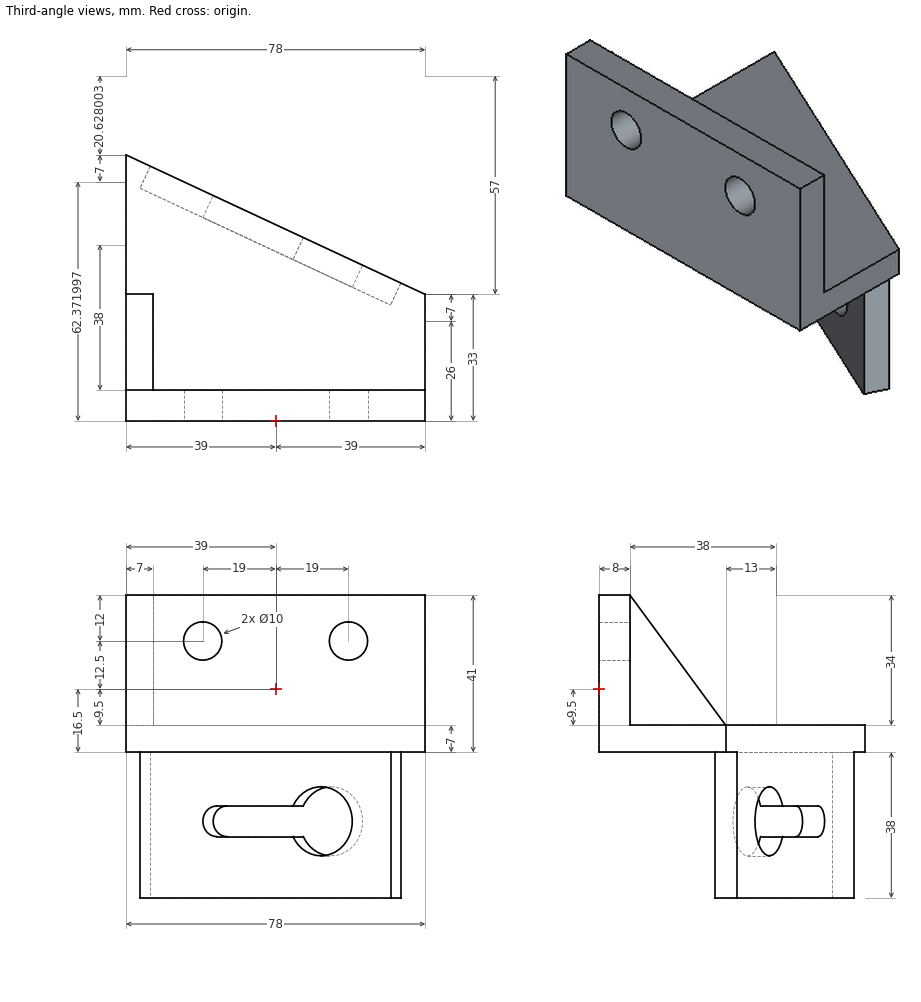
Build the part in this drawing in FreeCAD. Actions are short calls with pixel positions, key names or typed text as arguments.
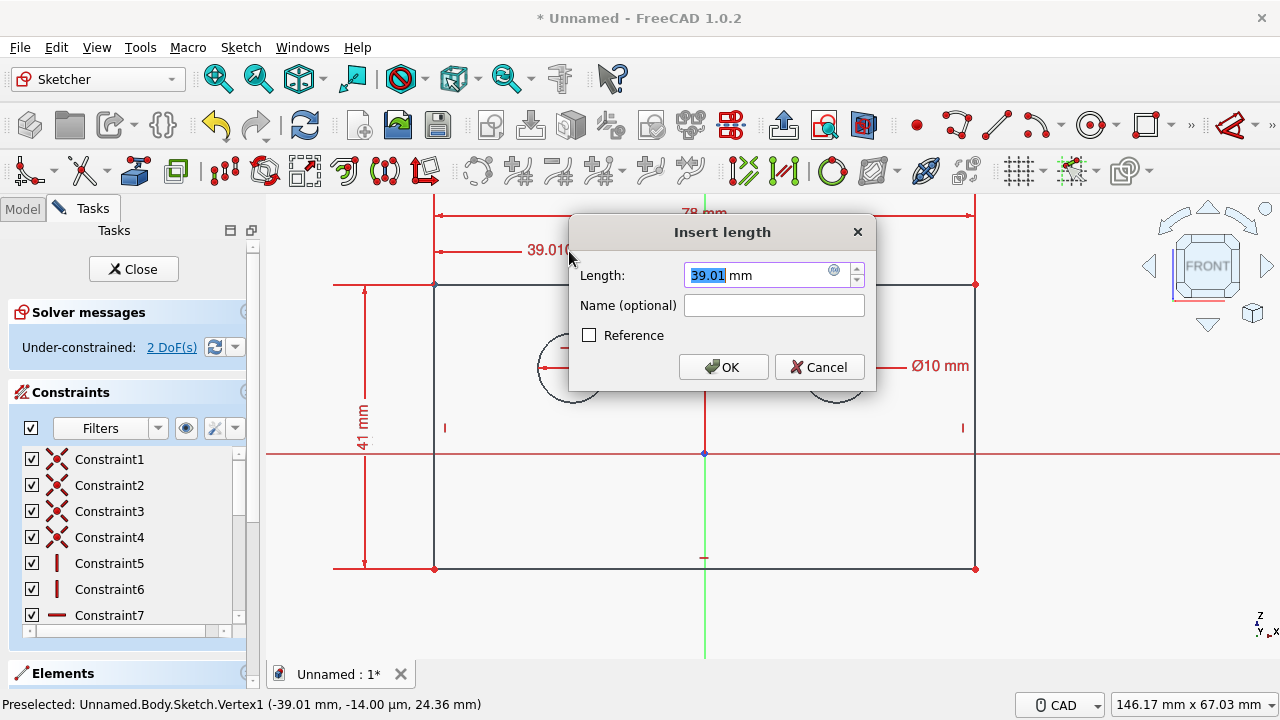
text(39)
key(Return)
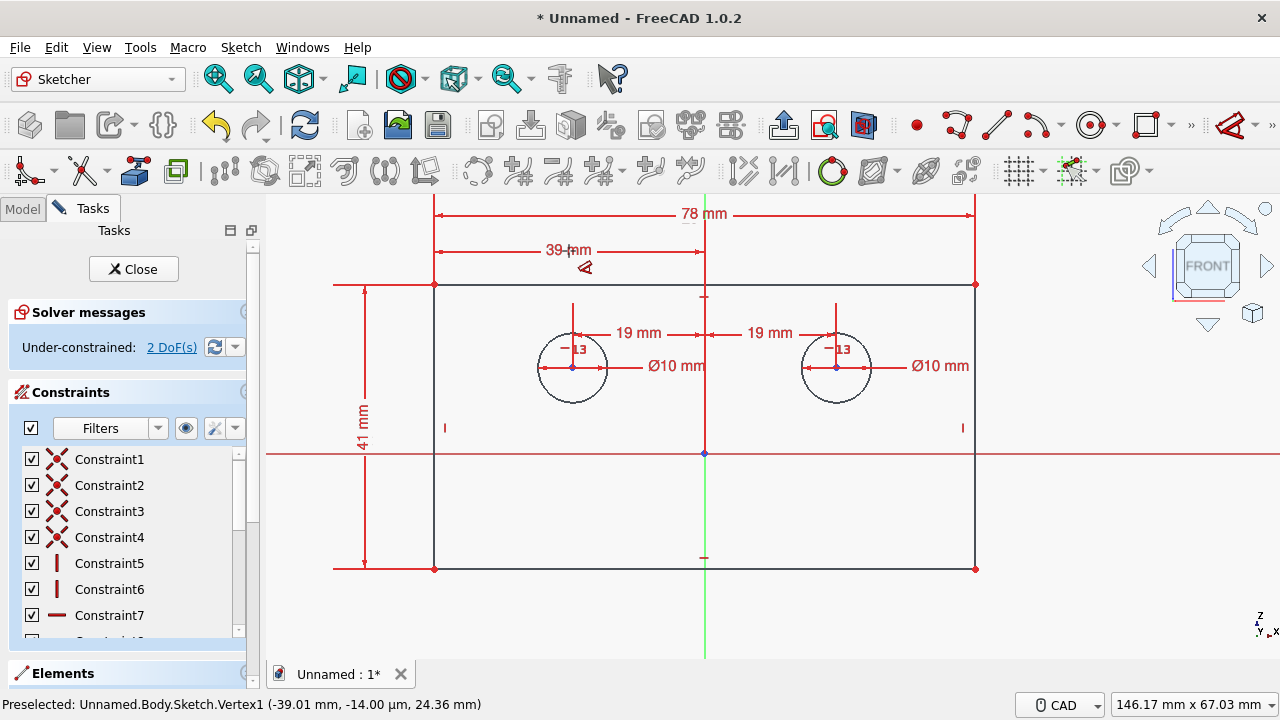
click(434, 285)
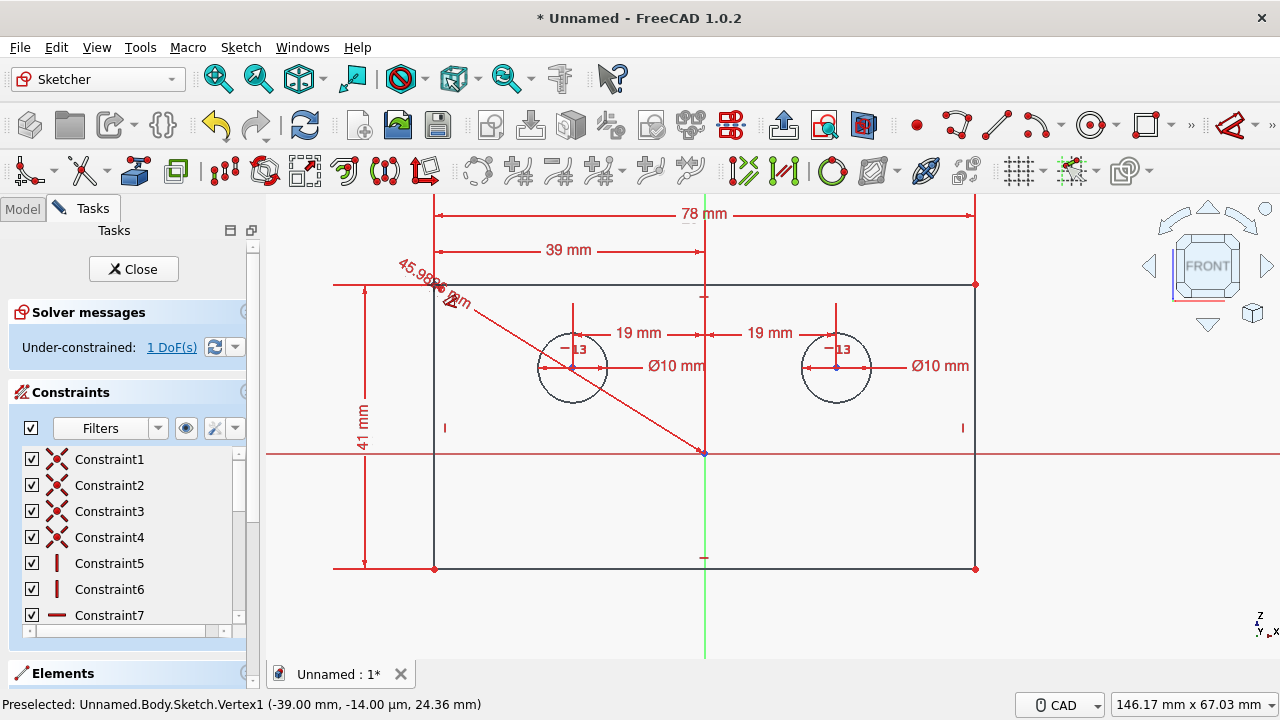
click(573, 368)
click(400, 327)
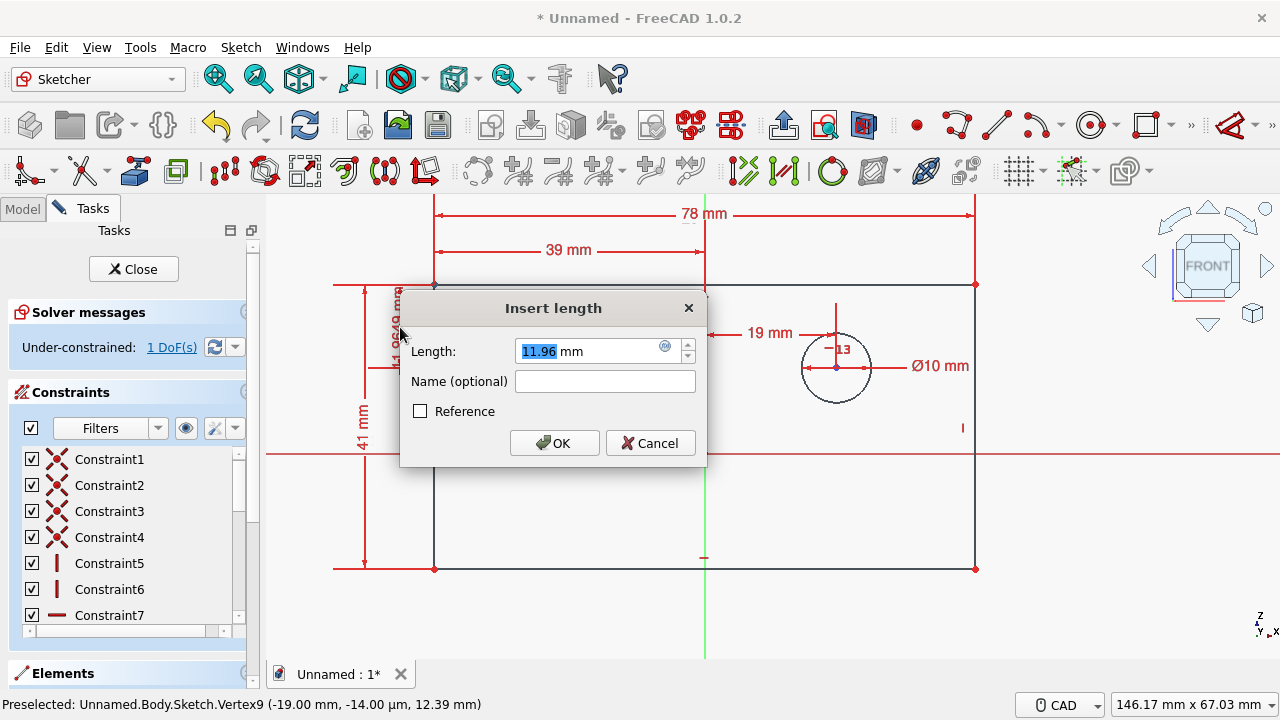
text(12)
key(Return)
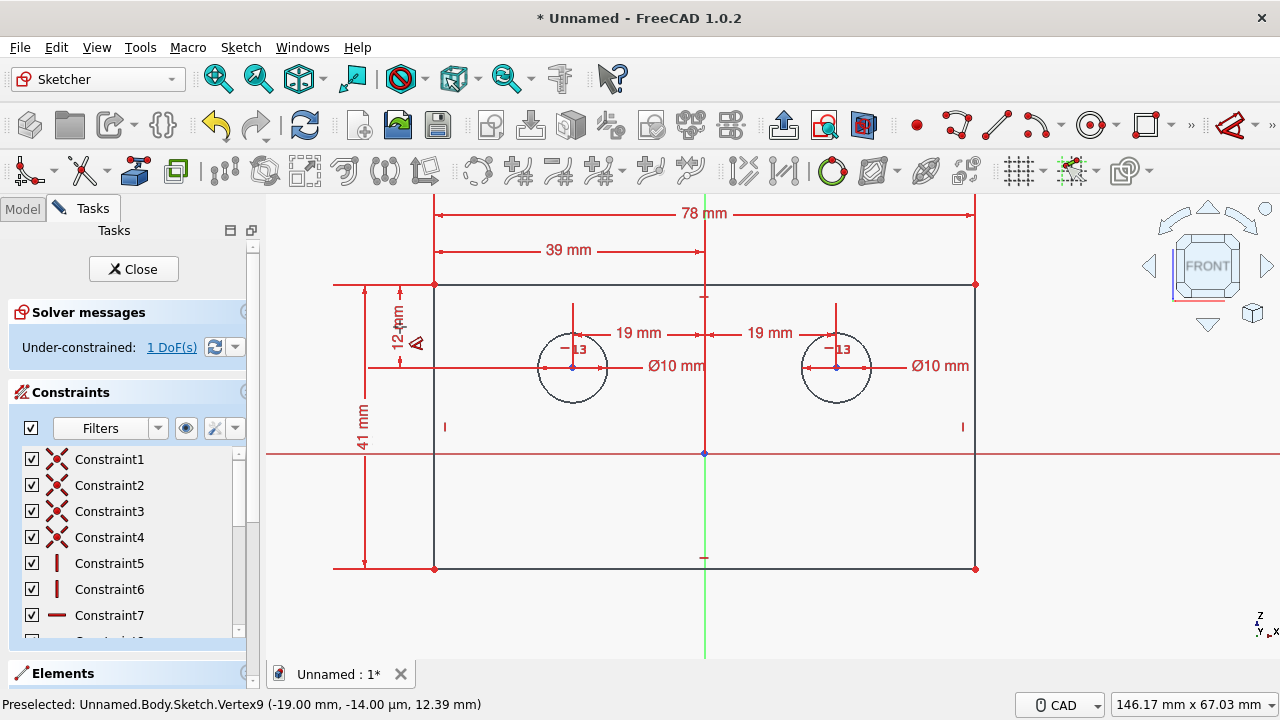
click(573, 368)
click(539, 411)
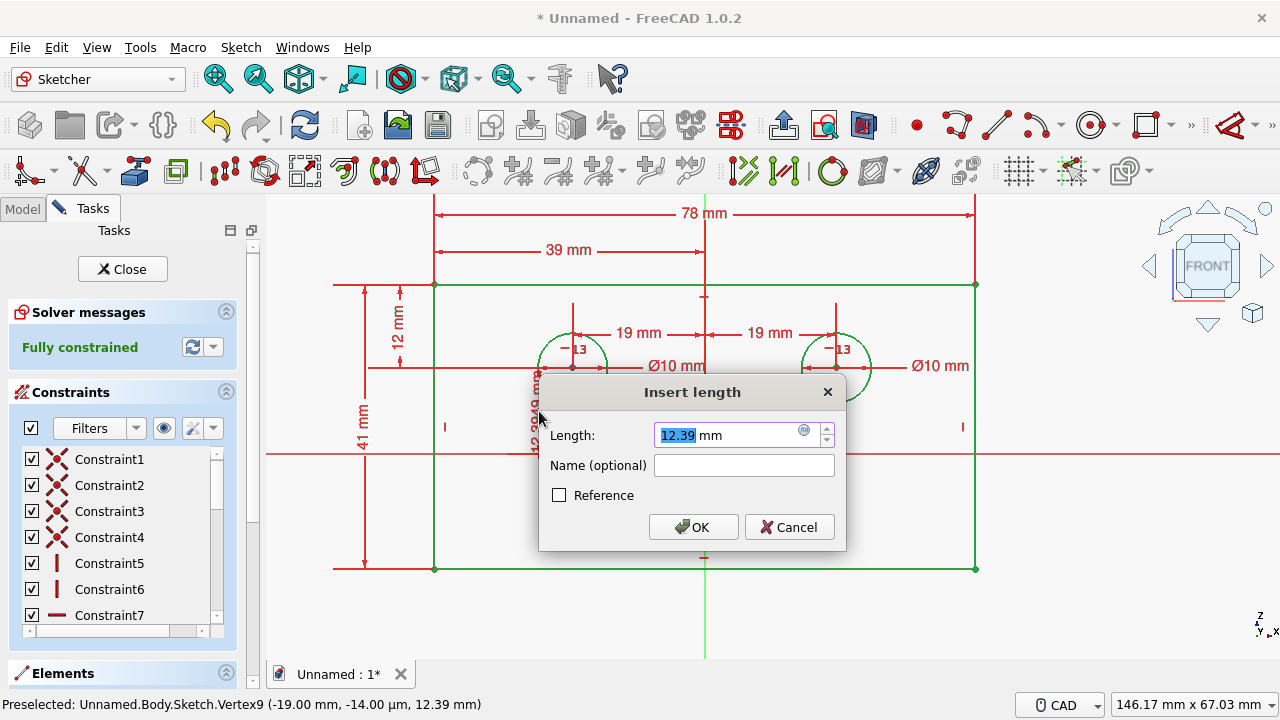
text(12.5)
key(Return)
key(Escape)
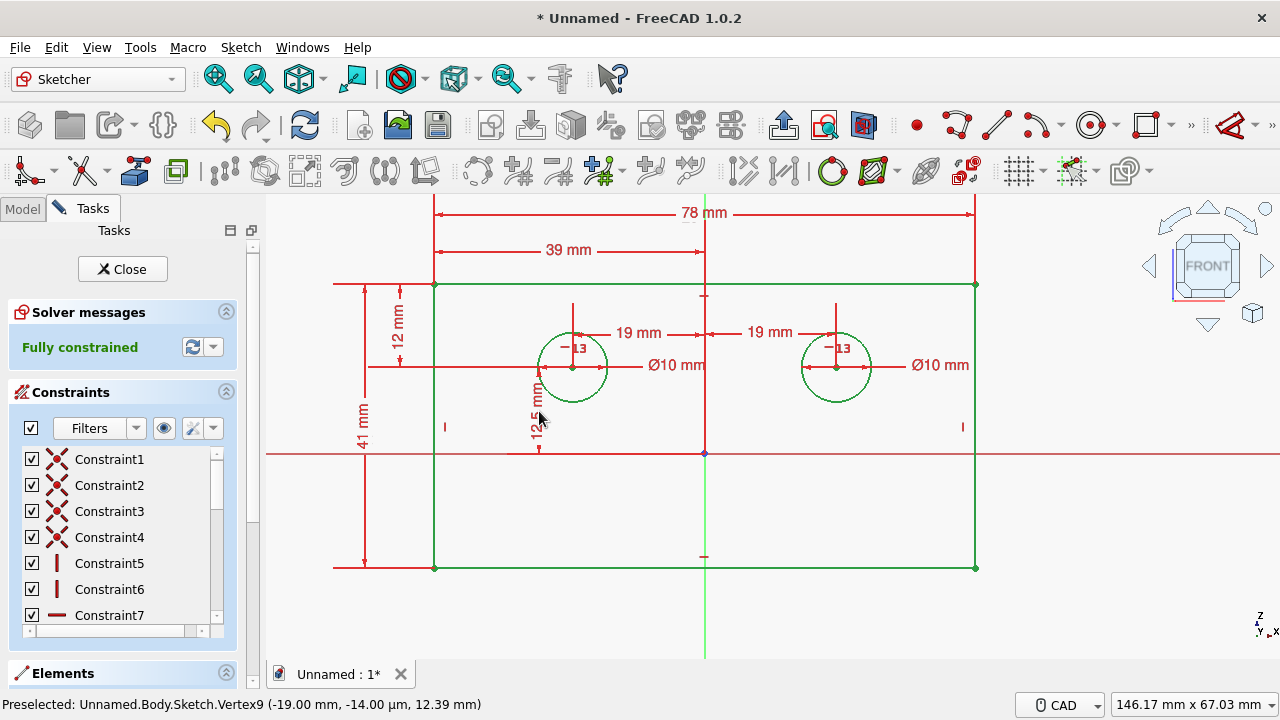
click(123, 269)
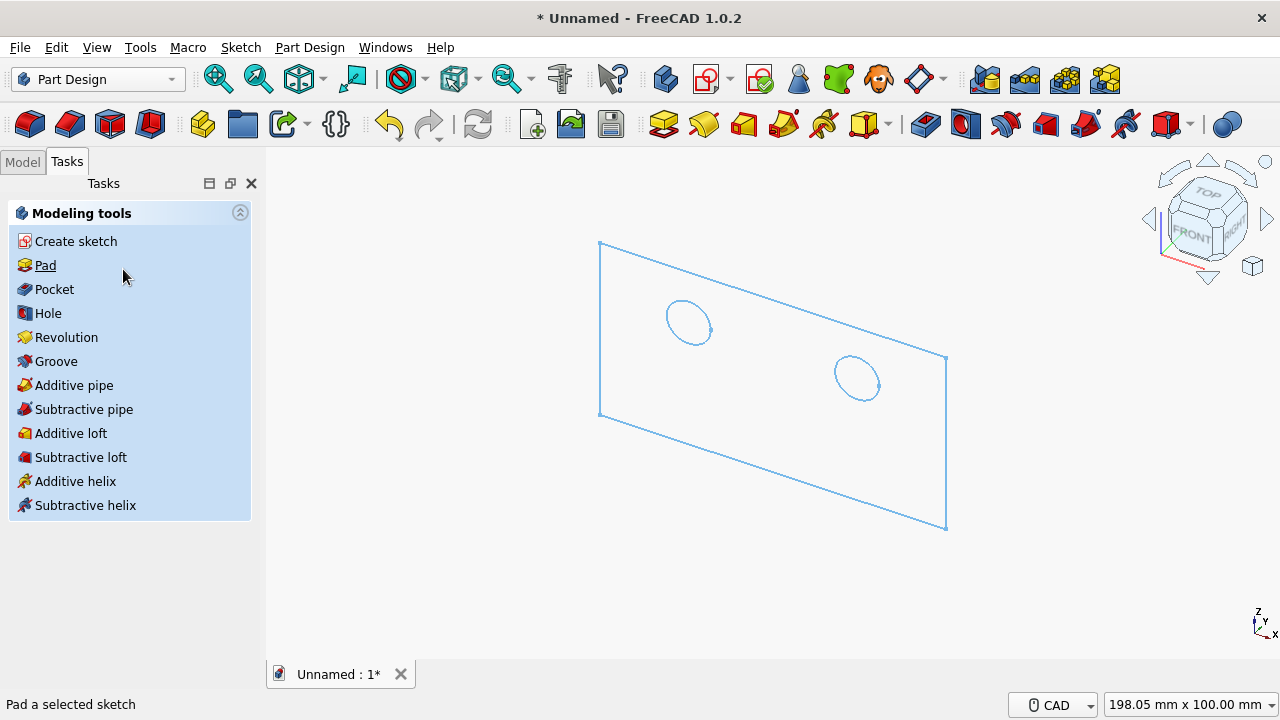
click(664, 124)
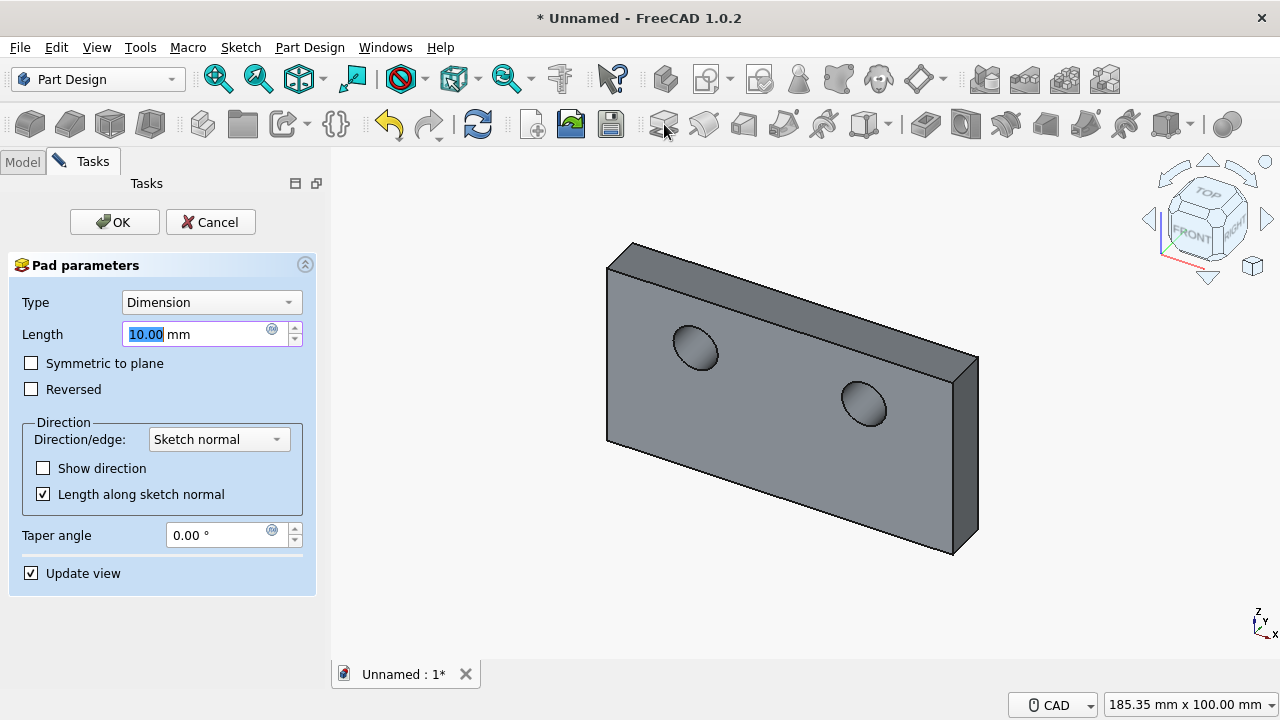
text(8)
key(Tab)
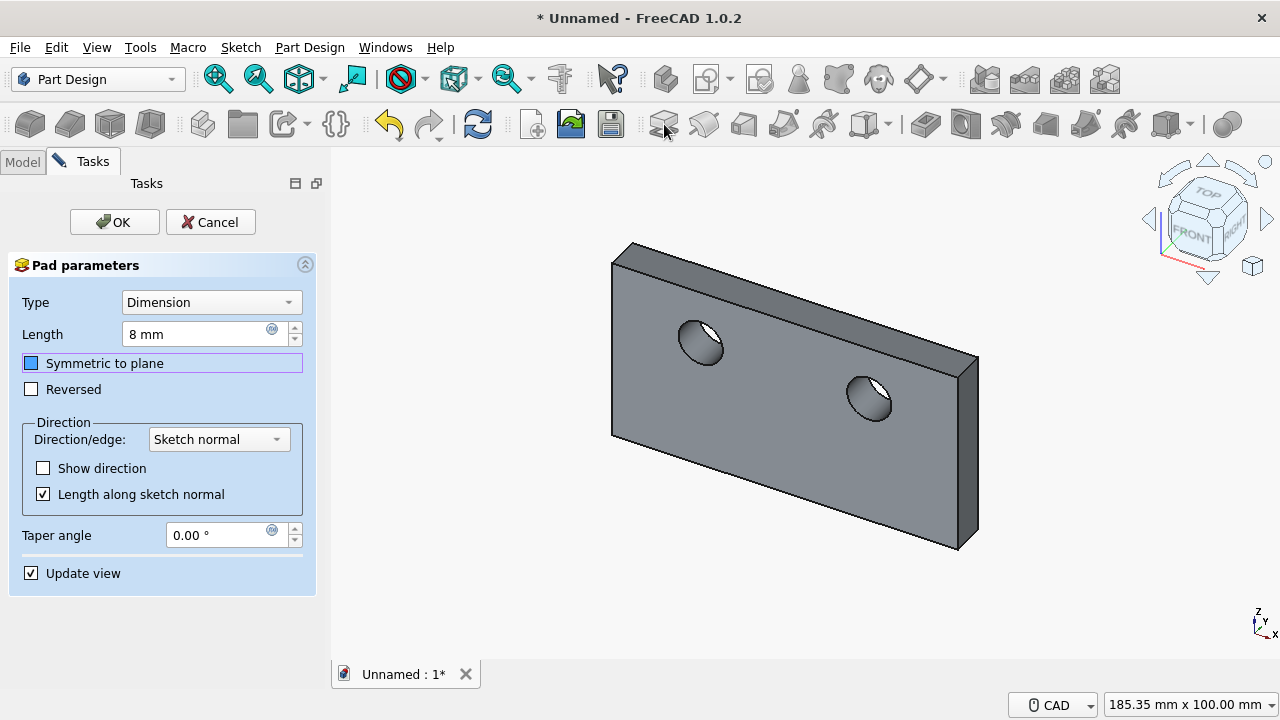
click(30, 389)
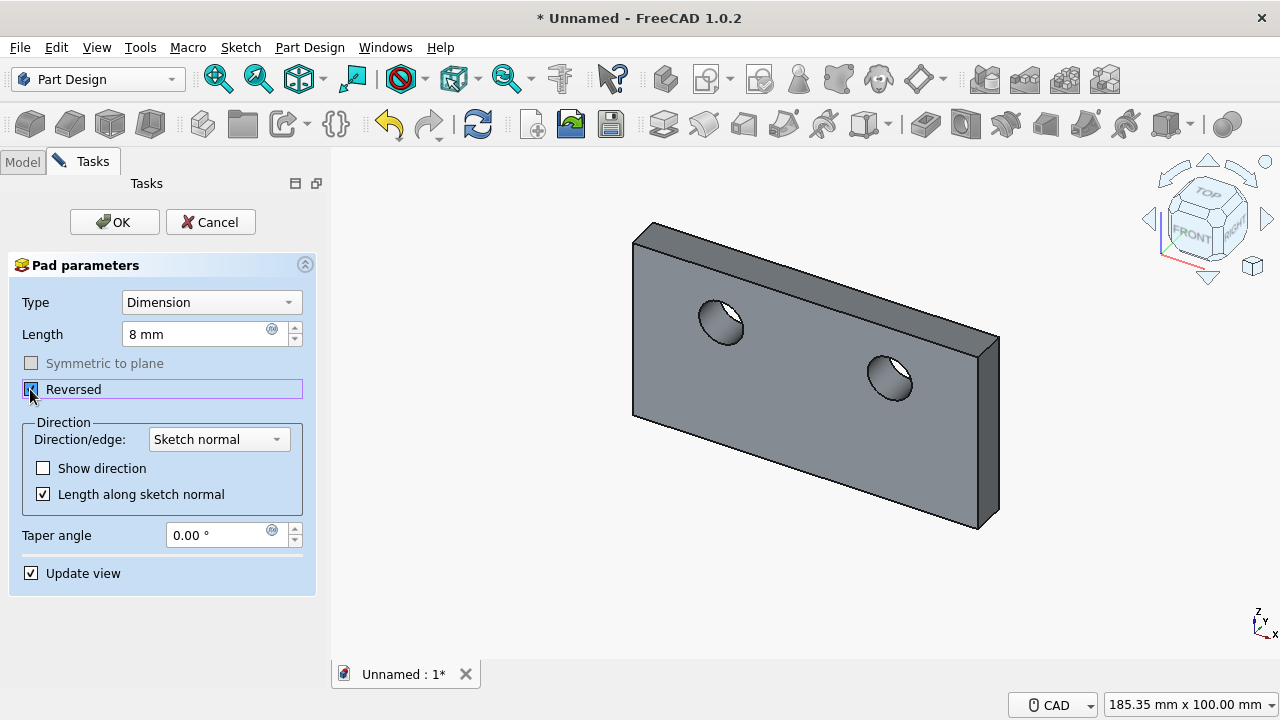
click(115, 222)